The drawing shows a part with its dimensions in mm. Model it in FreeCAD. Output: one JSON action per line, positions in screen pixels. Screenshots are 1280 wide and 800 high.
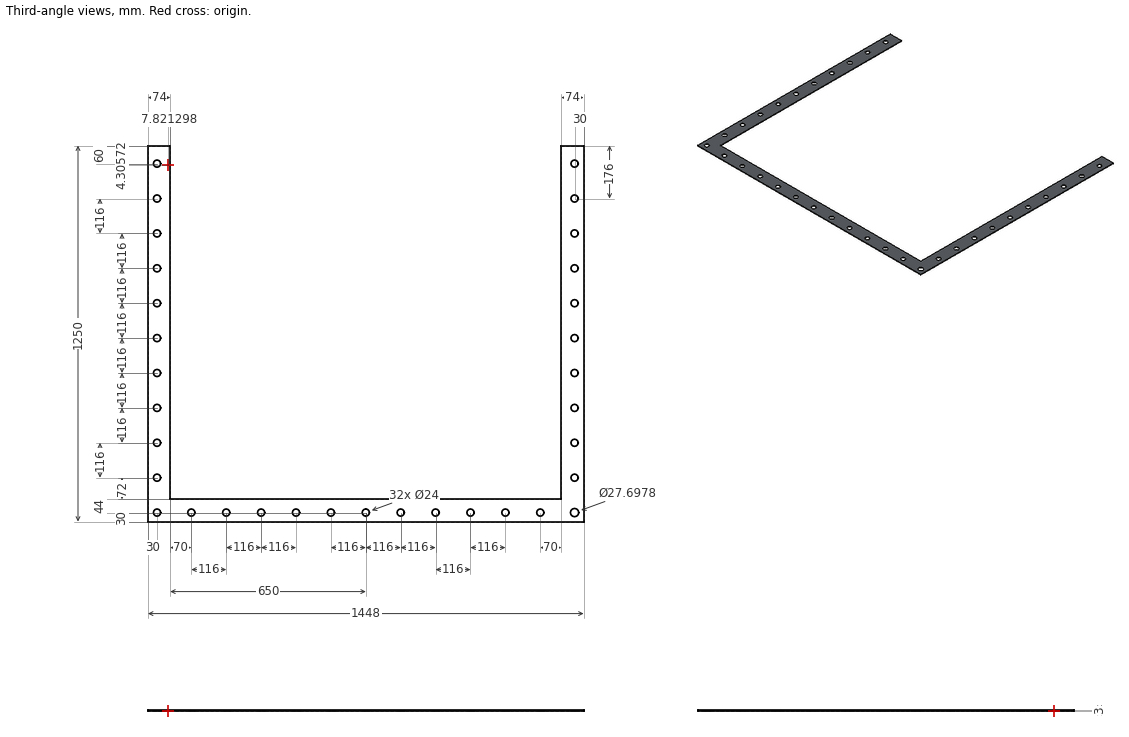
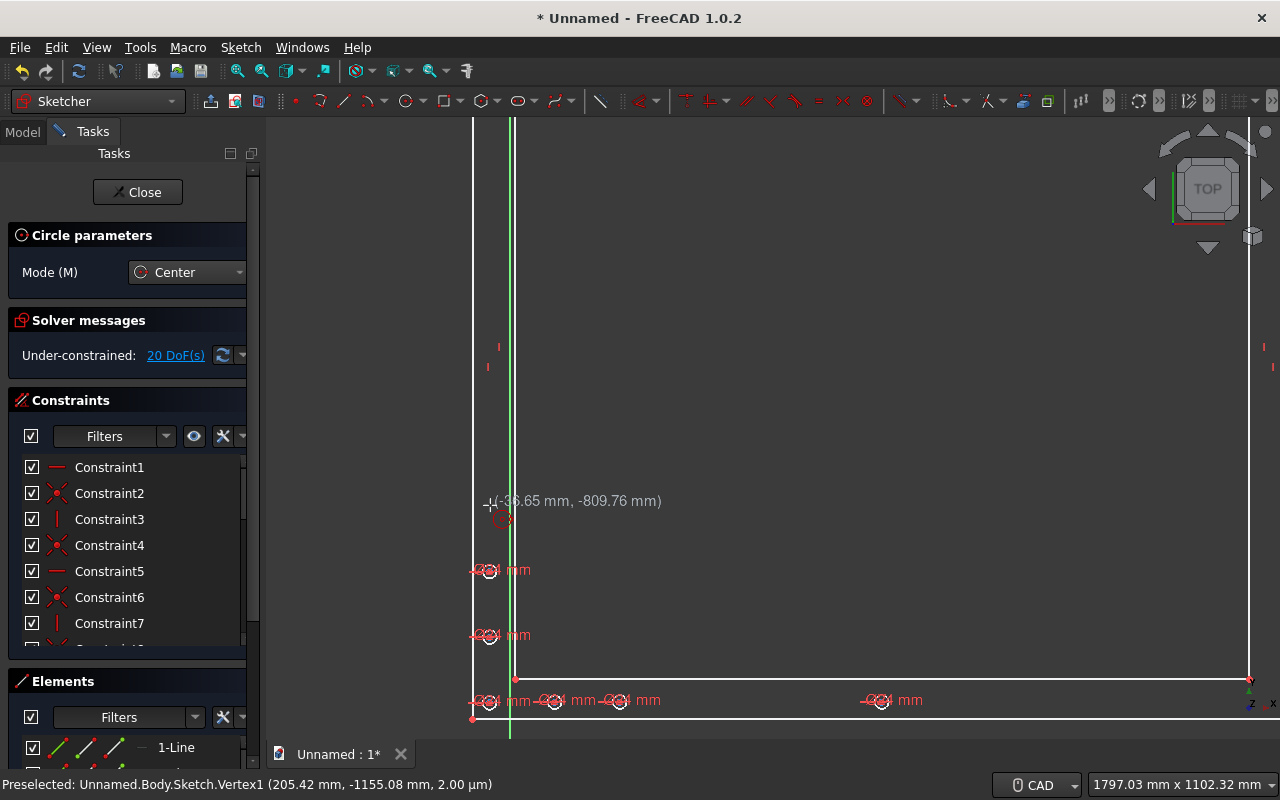
{"action": "left_click", "coordinate": [490, 505]}
{"action": "mouse_move", "coordinate": [495, 500]}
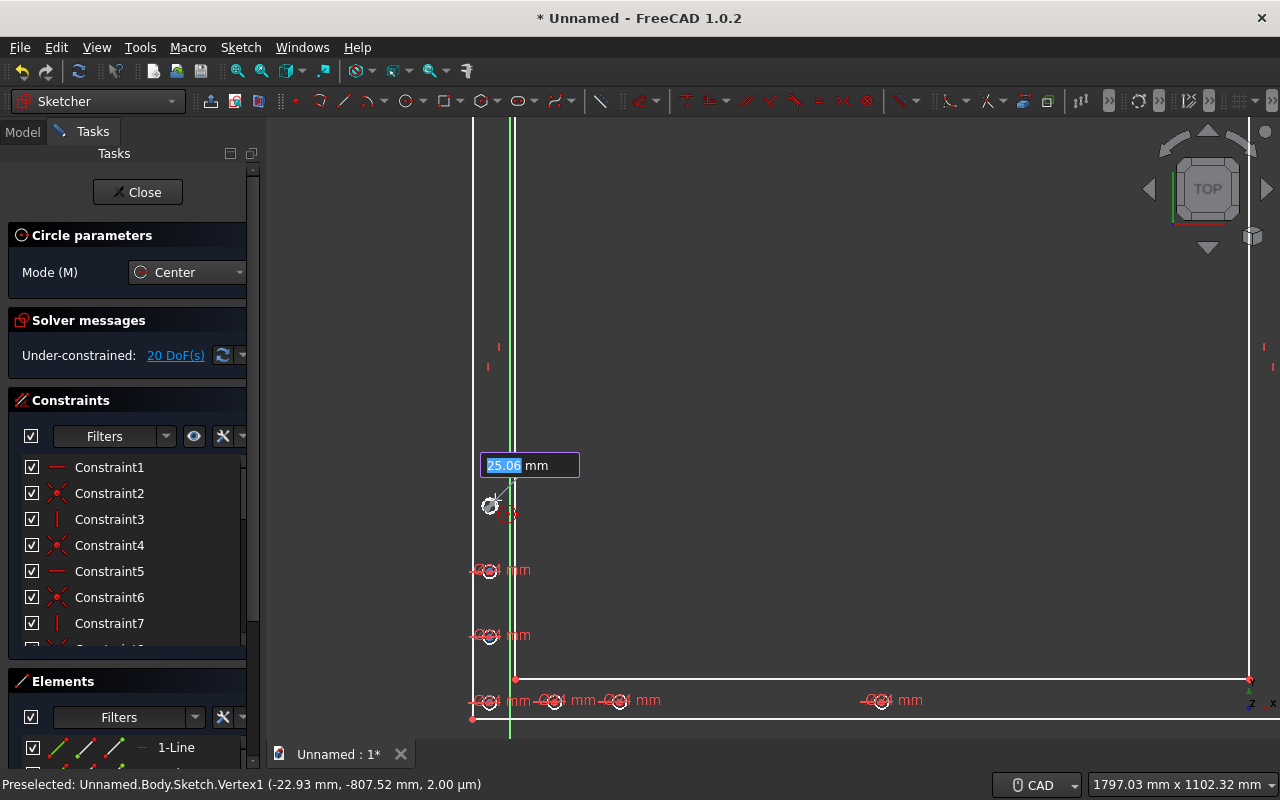
{"action": "type", "text": "24"}
{"action": "key", "text": "Return"}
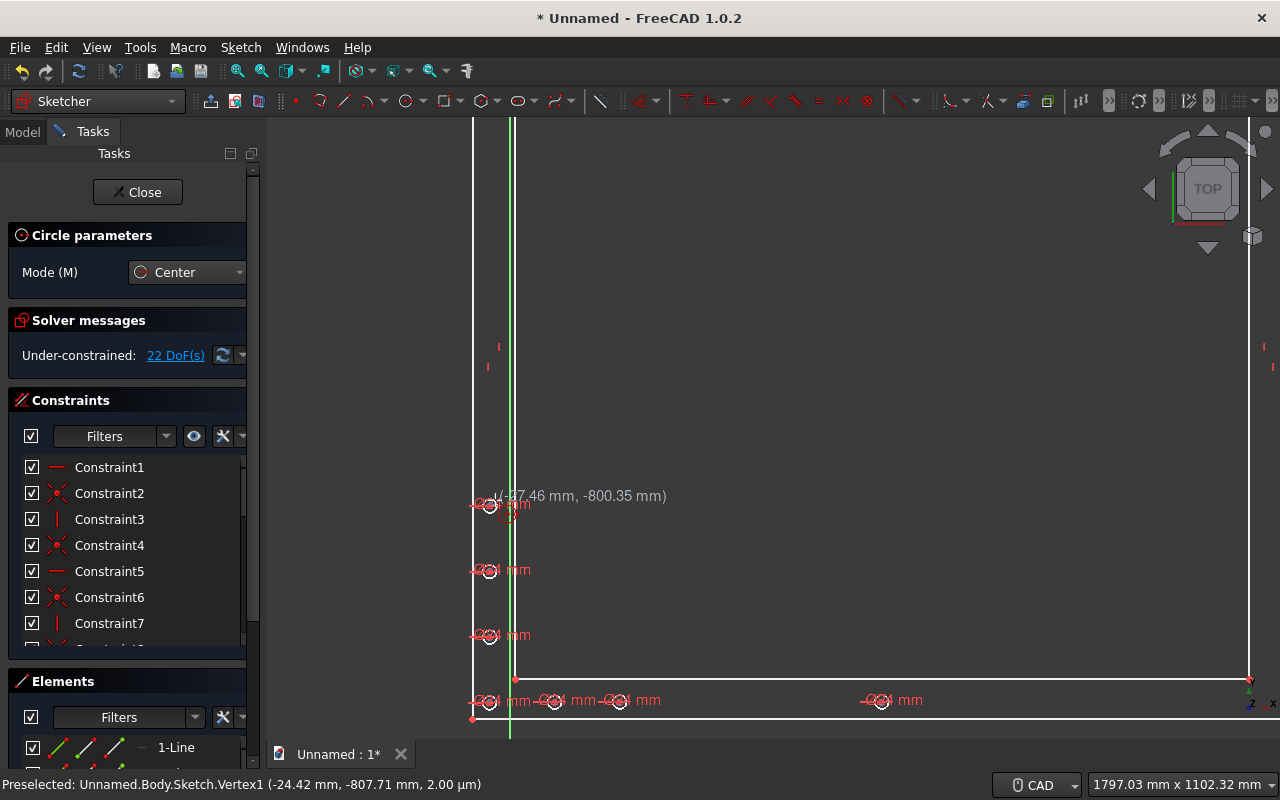
{"action": "scroll", "coordinate": [490, 440], "scroll_direction": "up", "scroll_amount": 7}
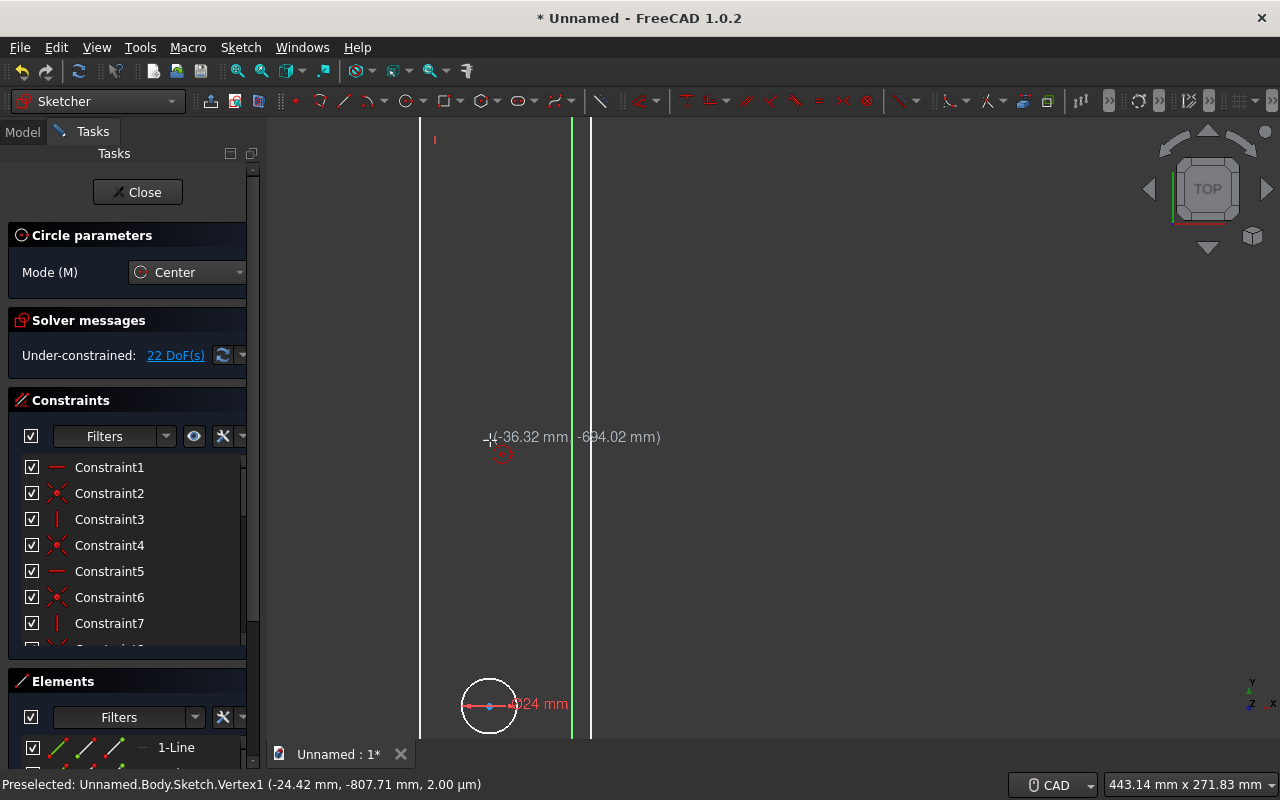
{"action": "scroll", "coordinate": [490, 473], "scroll_direction": "down", "scroll_amount": 10}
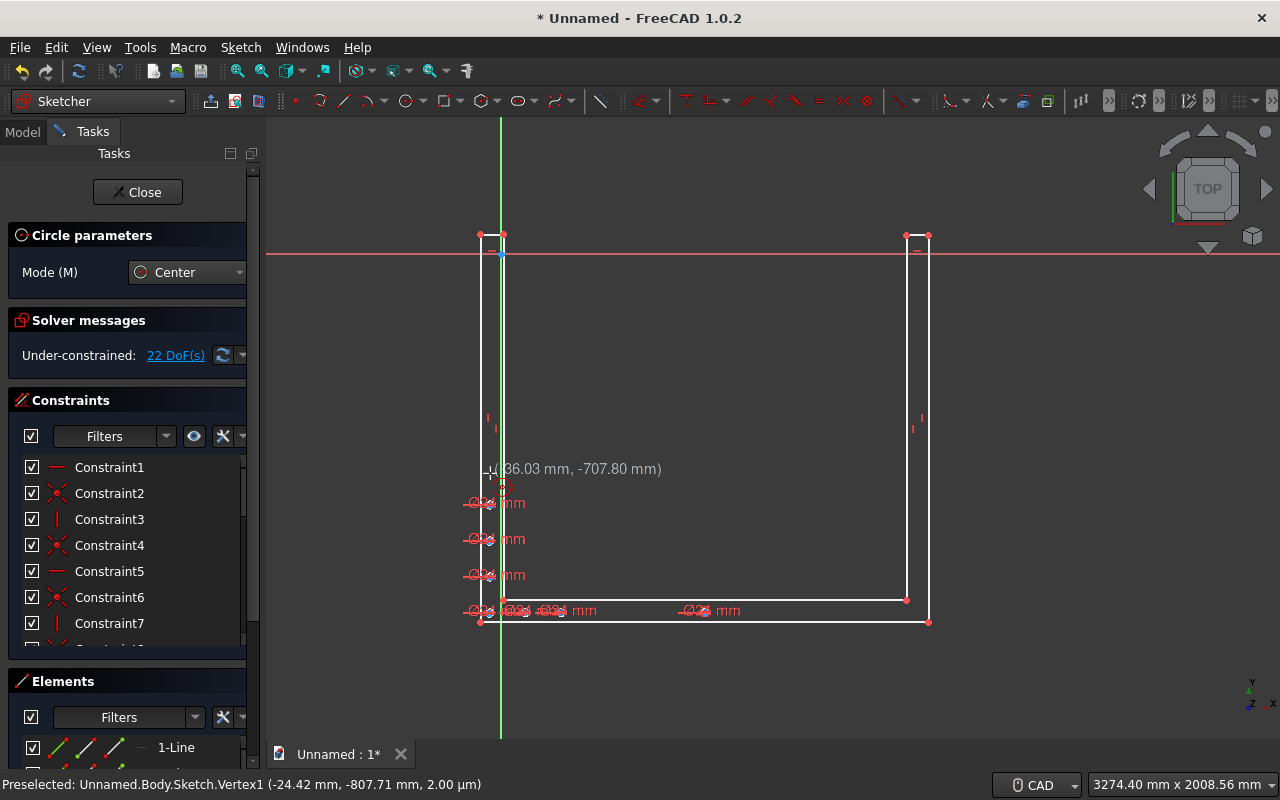
{"action": "scroll", "coordinate": [490, 469], "scroll_direction": "up", "scroll_amount": 3}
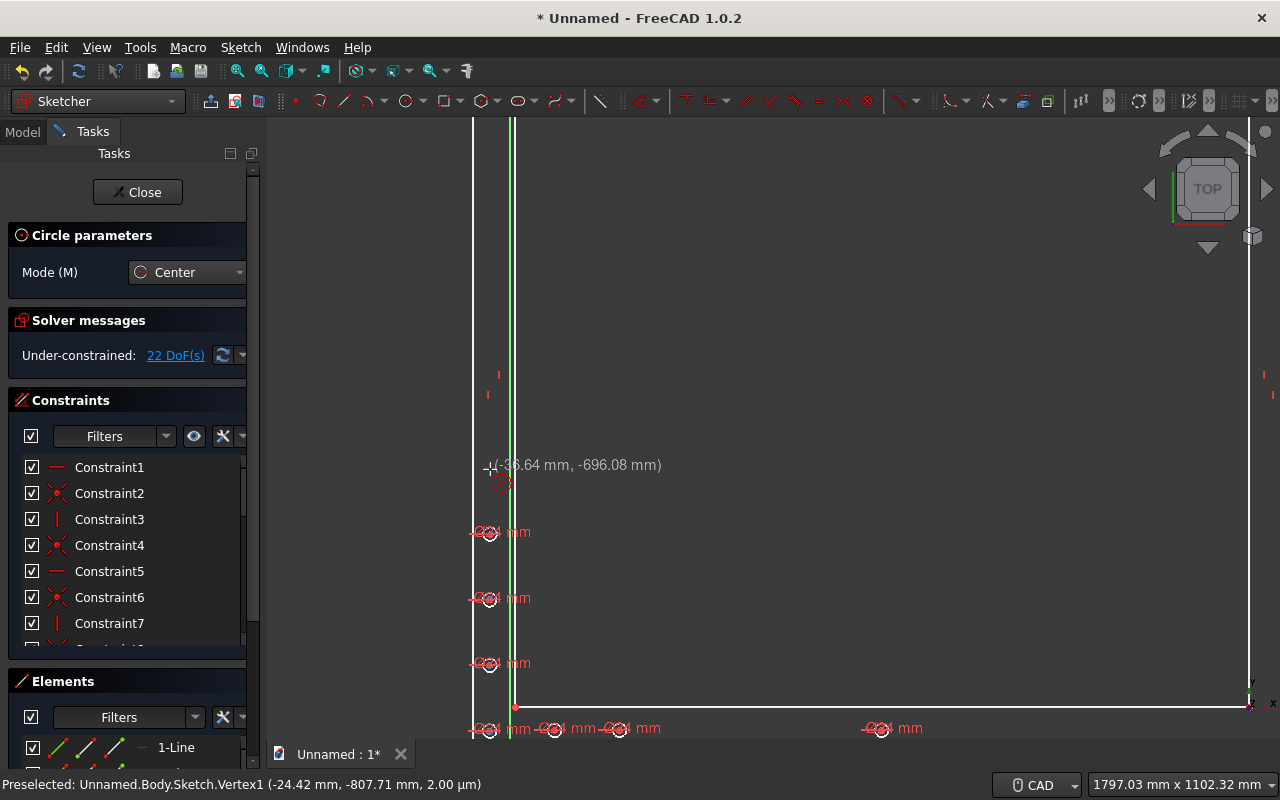
{"action": "left_click", "coordinate": [490, 468]}
{"action": "mouse_move", "coordinate": [495, 463]}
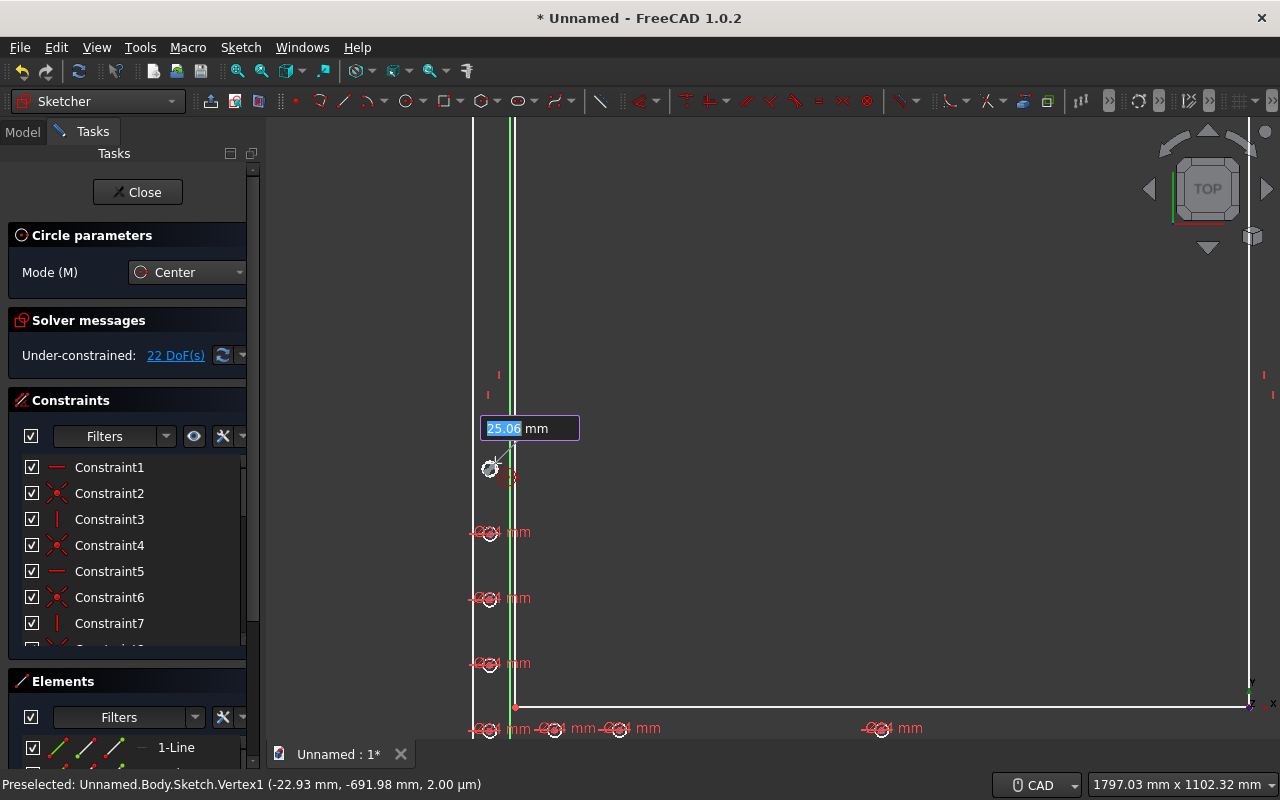
{"action": "type", "text": "24"}
{"action": "key", "text": "Return"}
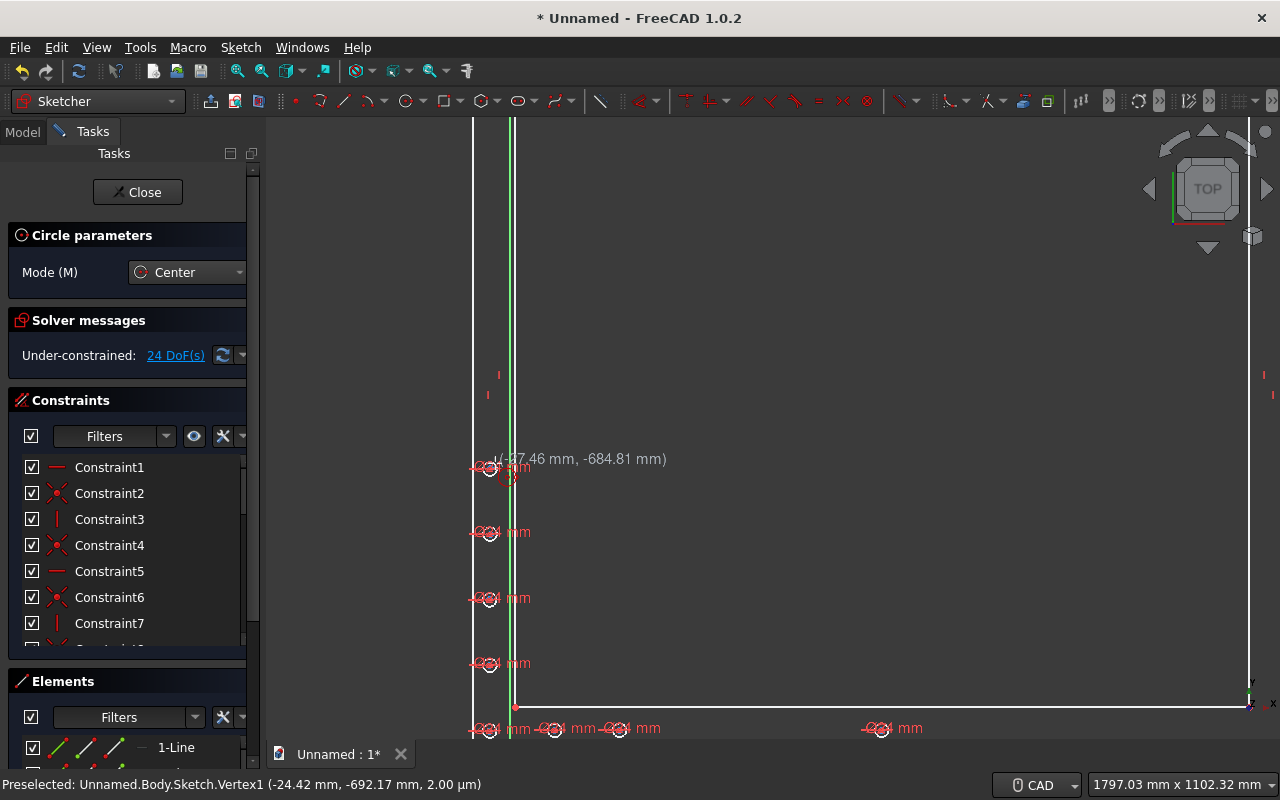
{"action": "scroll", "coordinate": [489, 469], "scroll_direction": "down", "scroll_amount": 3}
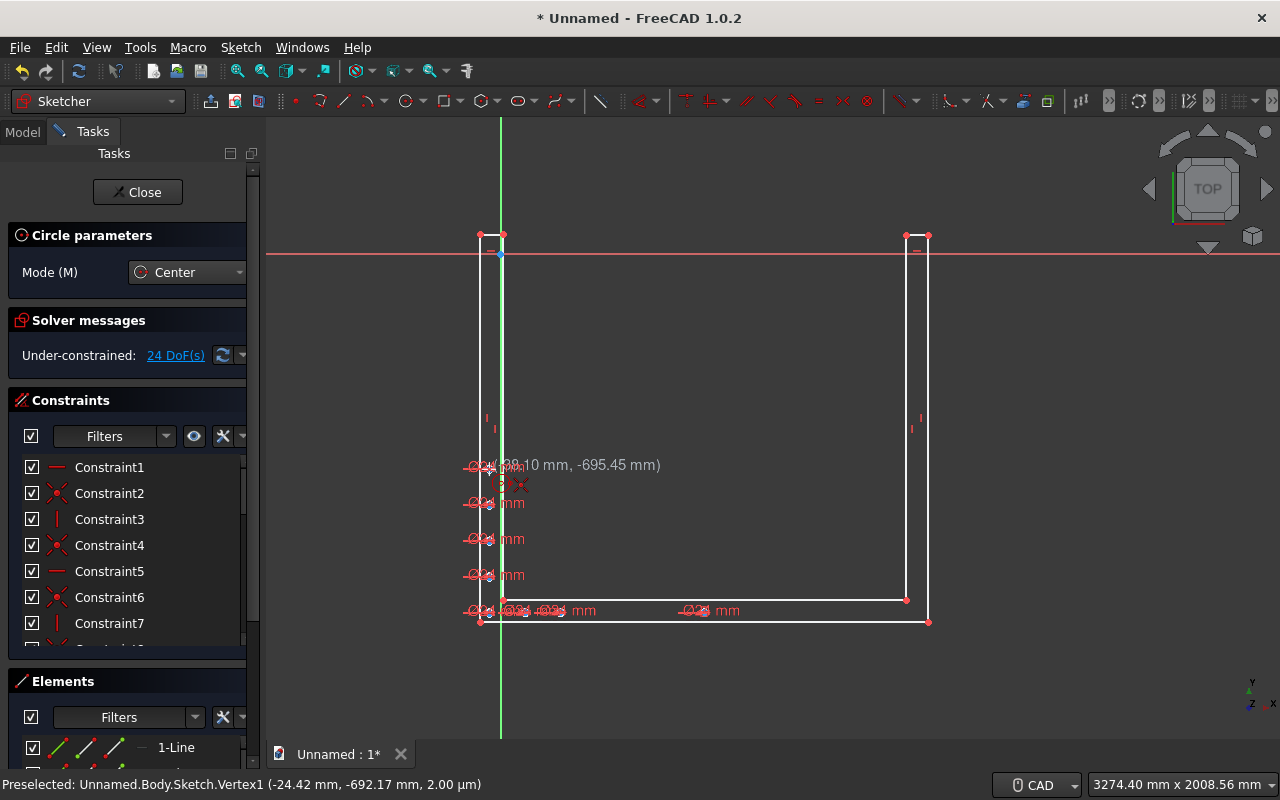
{"action": "scroll", "coordinate": [597, 612], "scroll_direction": "up", "scroll_amount": 10}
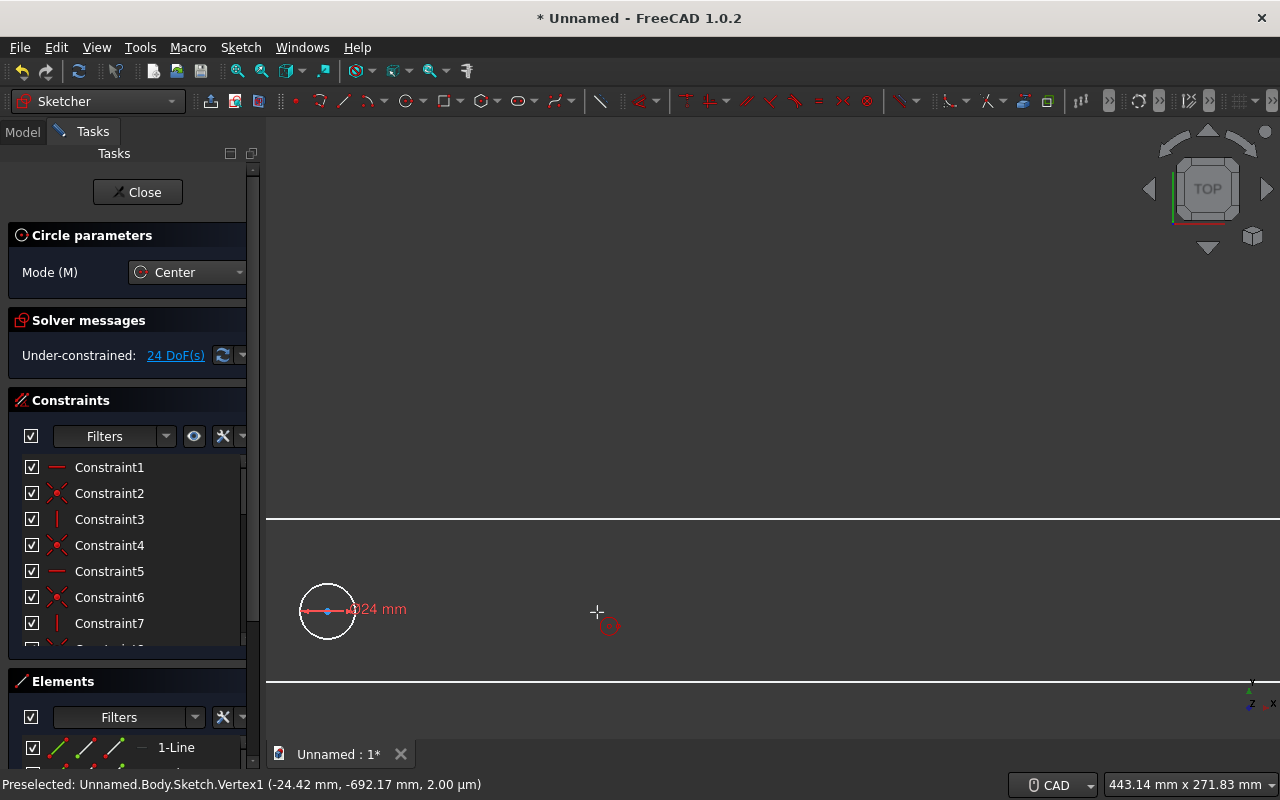
{"action": "scroll", "coordinate": [597, 613], "scroll_direction": "down", "scroll_amount": 10}